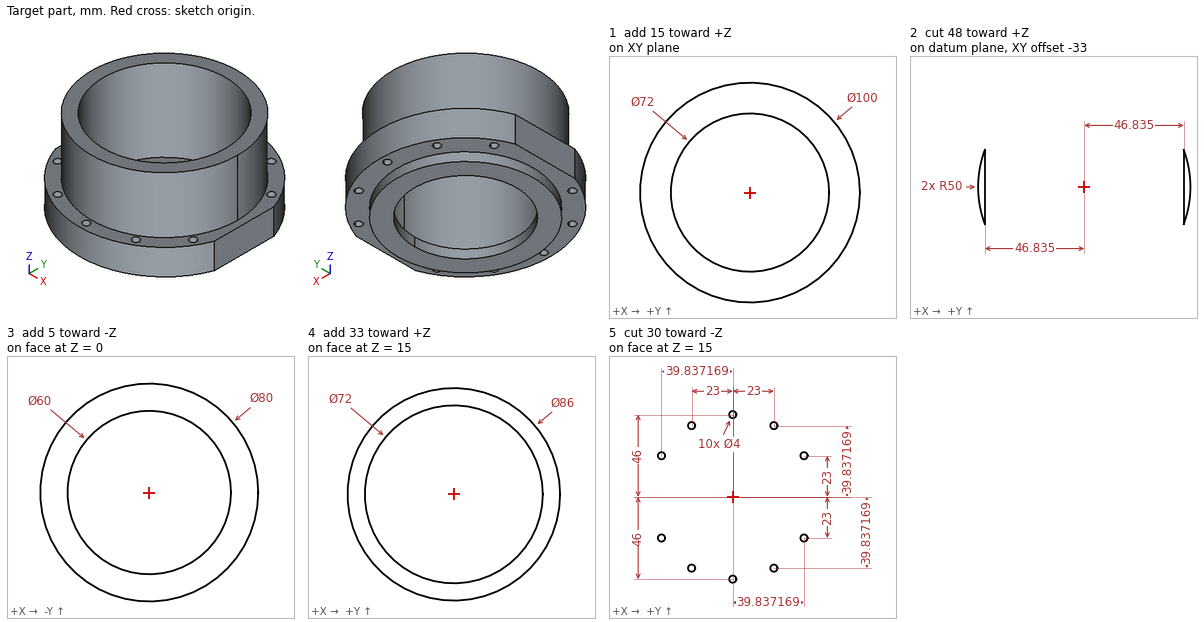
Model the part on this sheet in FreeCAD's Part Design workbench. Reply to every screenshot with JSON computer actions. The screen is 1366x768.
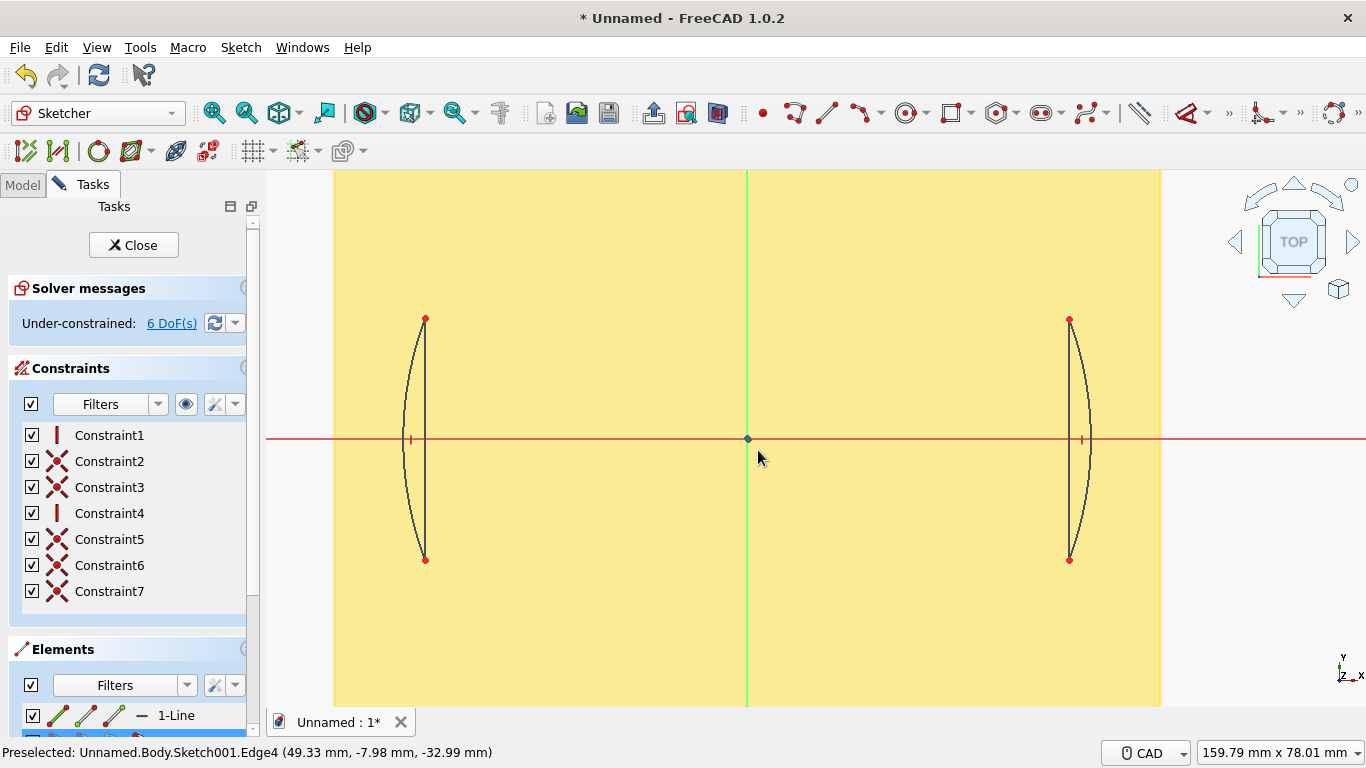
{"action": "key", "text": "c"}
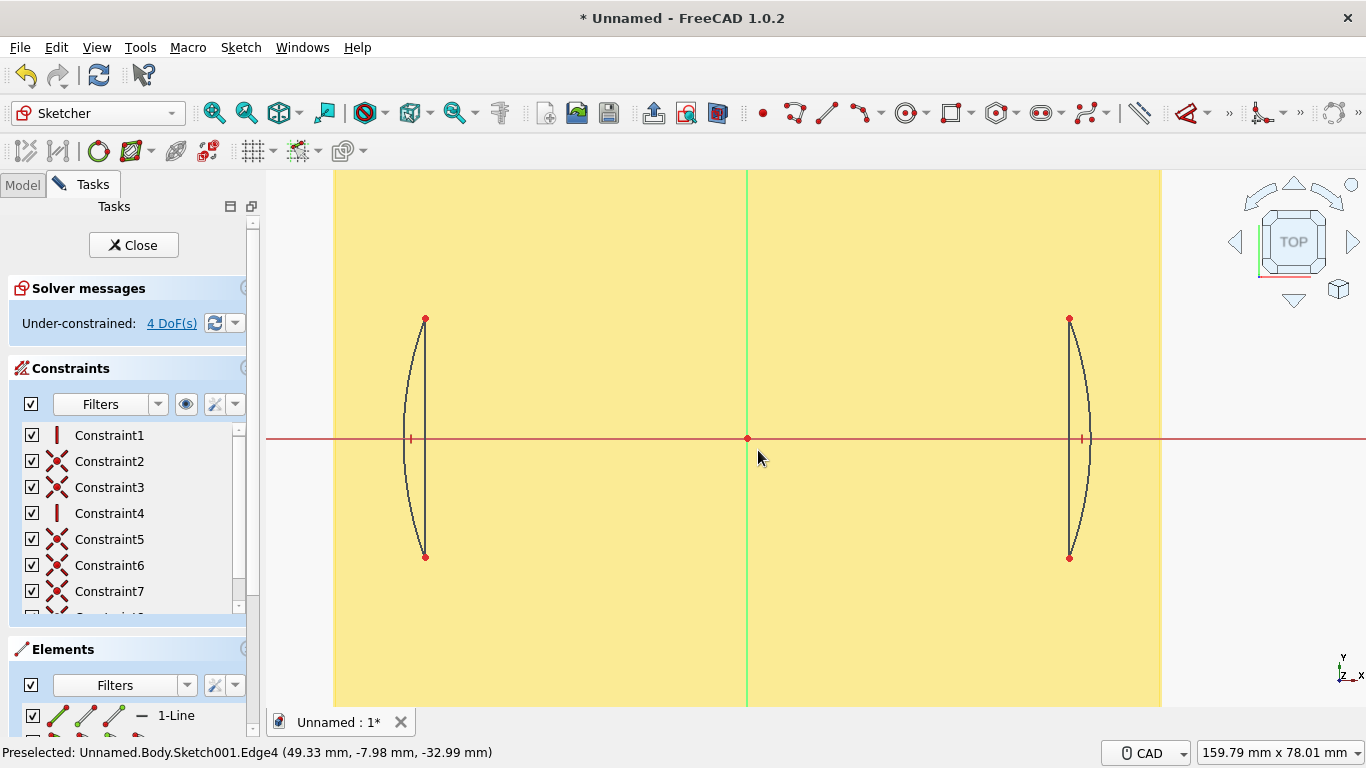
{"action": "left_click", "coordinate": [407, 390]}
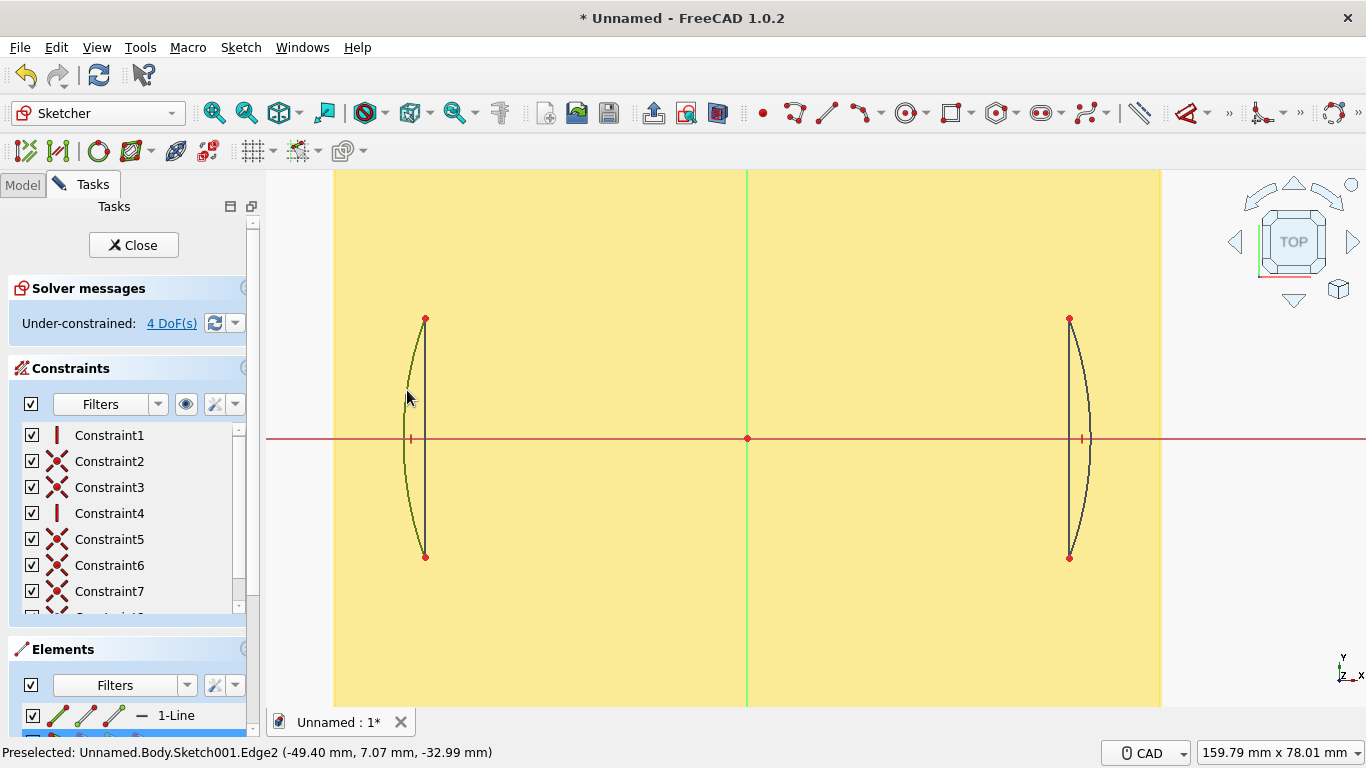
{"action": "left_click", "coordinate": [1087, 487]}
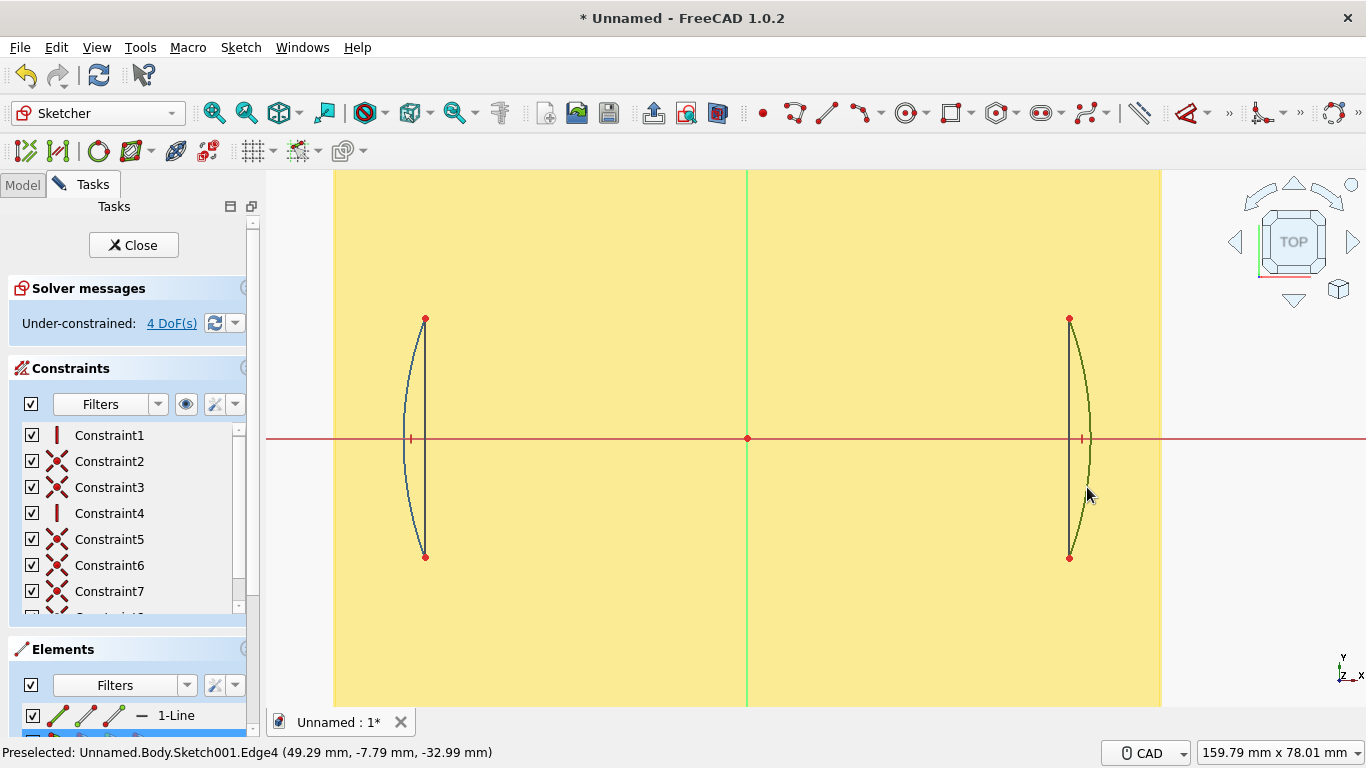
{"action": "key", "text": "e"}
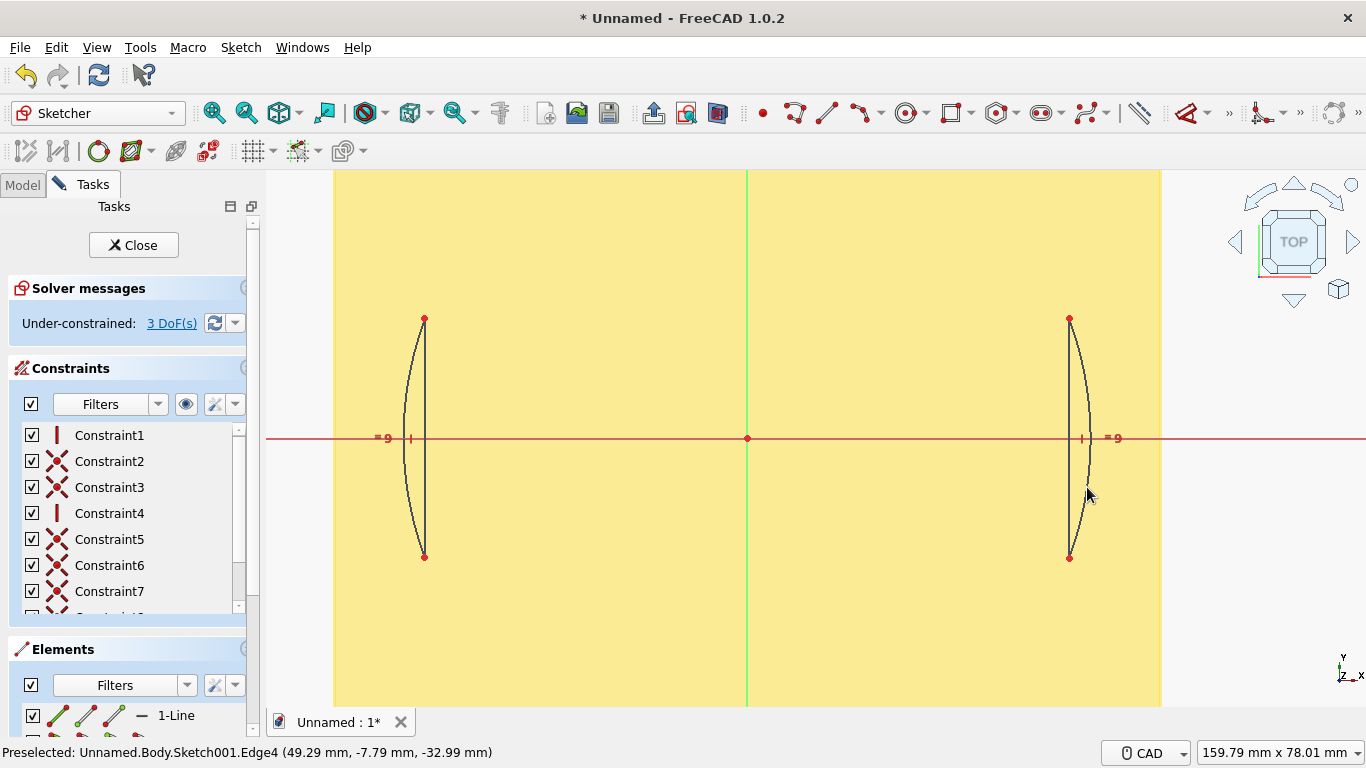
{"action": "left_click", "coordinate": [1186, 114]}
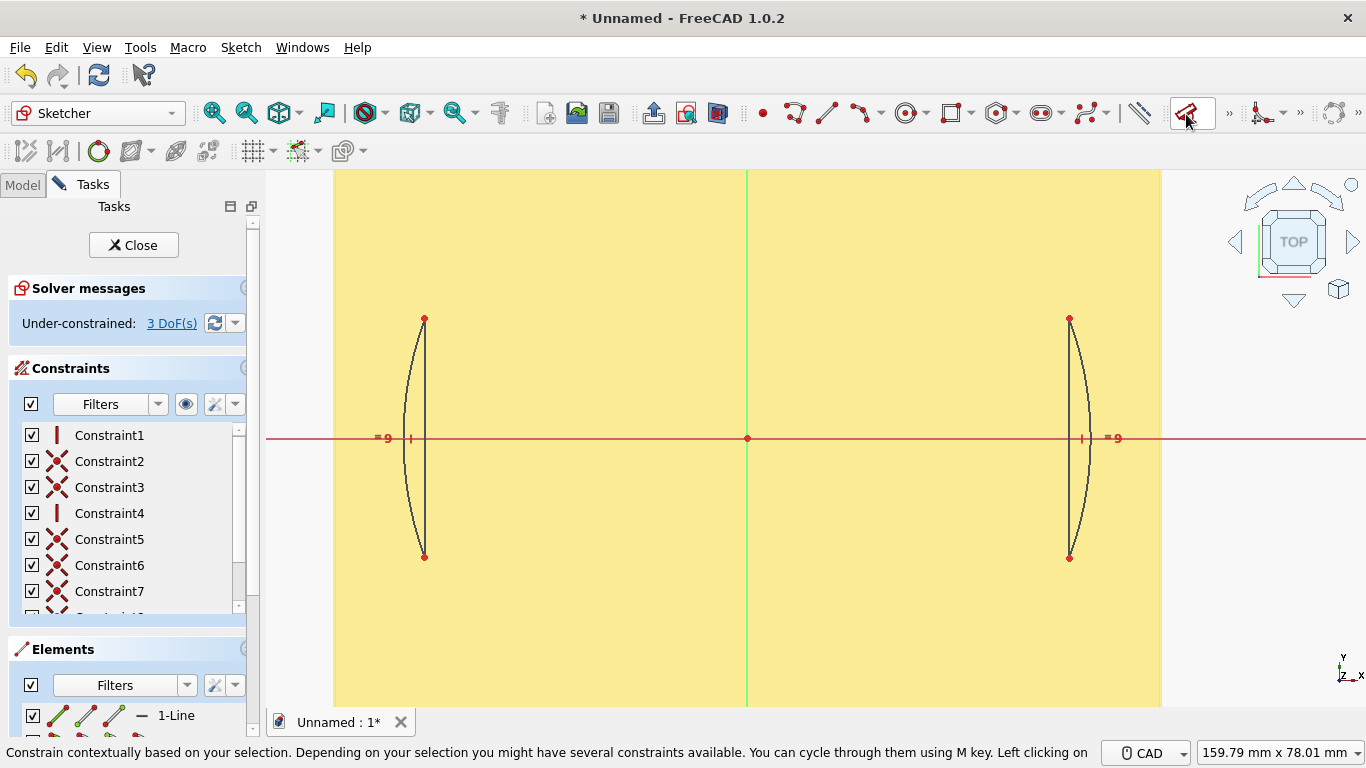
{"action": "left_click", "coordinate": [407, 390]}
{"action": "left_click", "coordinate": [375, 385]}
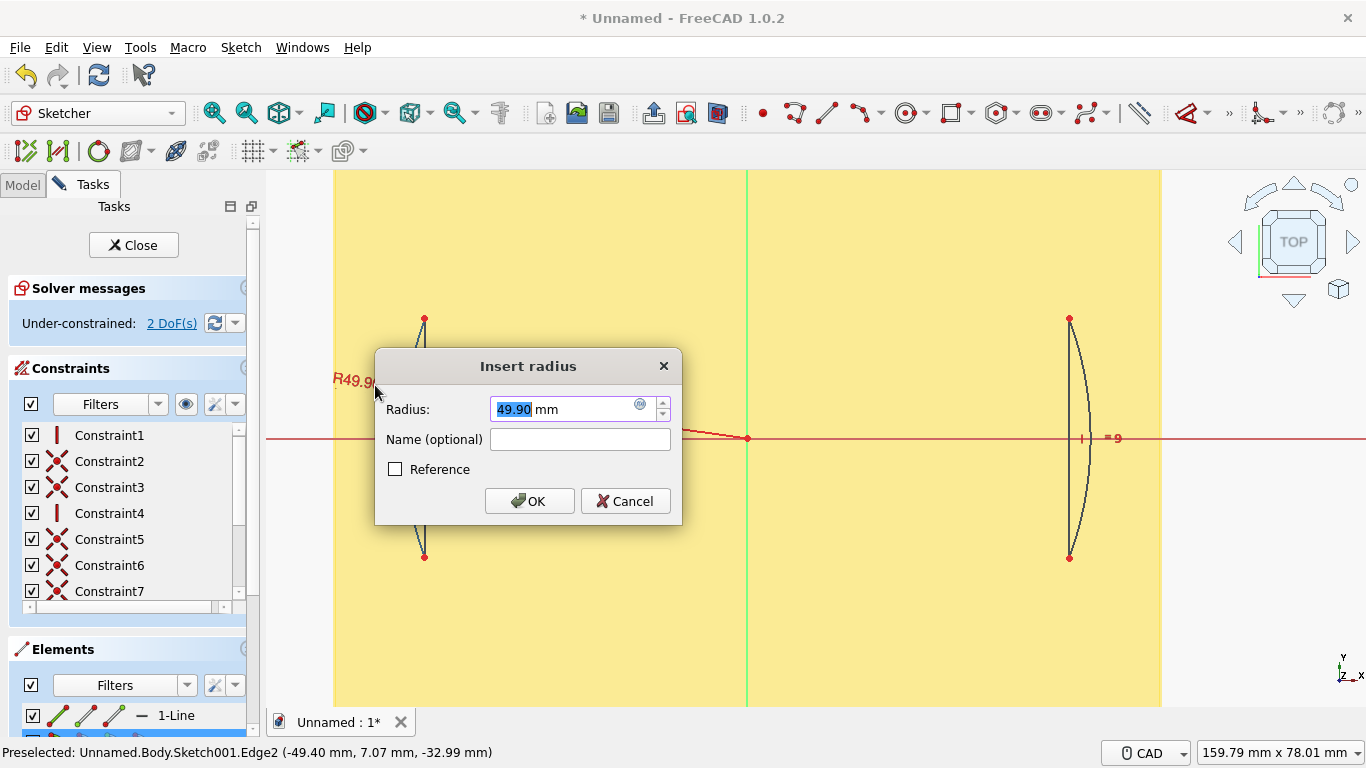
{"action": "type", "text": "50"}
{"action": "key", "text": "Return"}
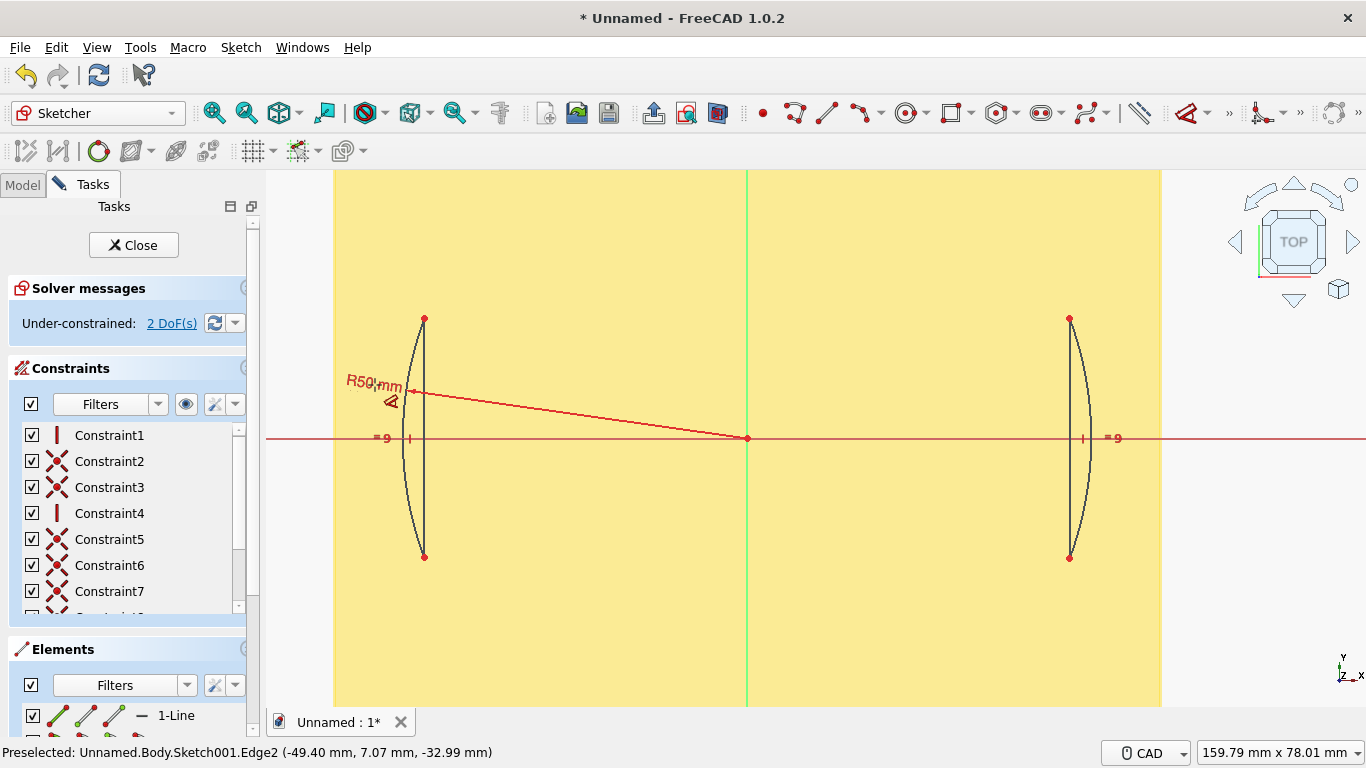
{"action": "left_click", "coordinate": [424, 558]}
{"action": "left_click", "coordinate": [586, 592]}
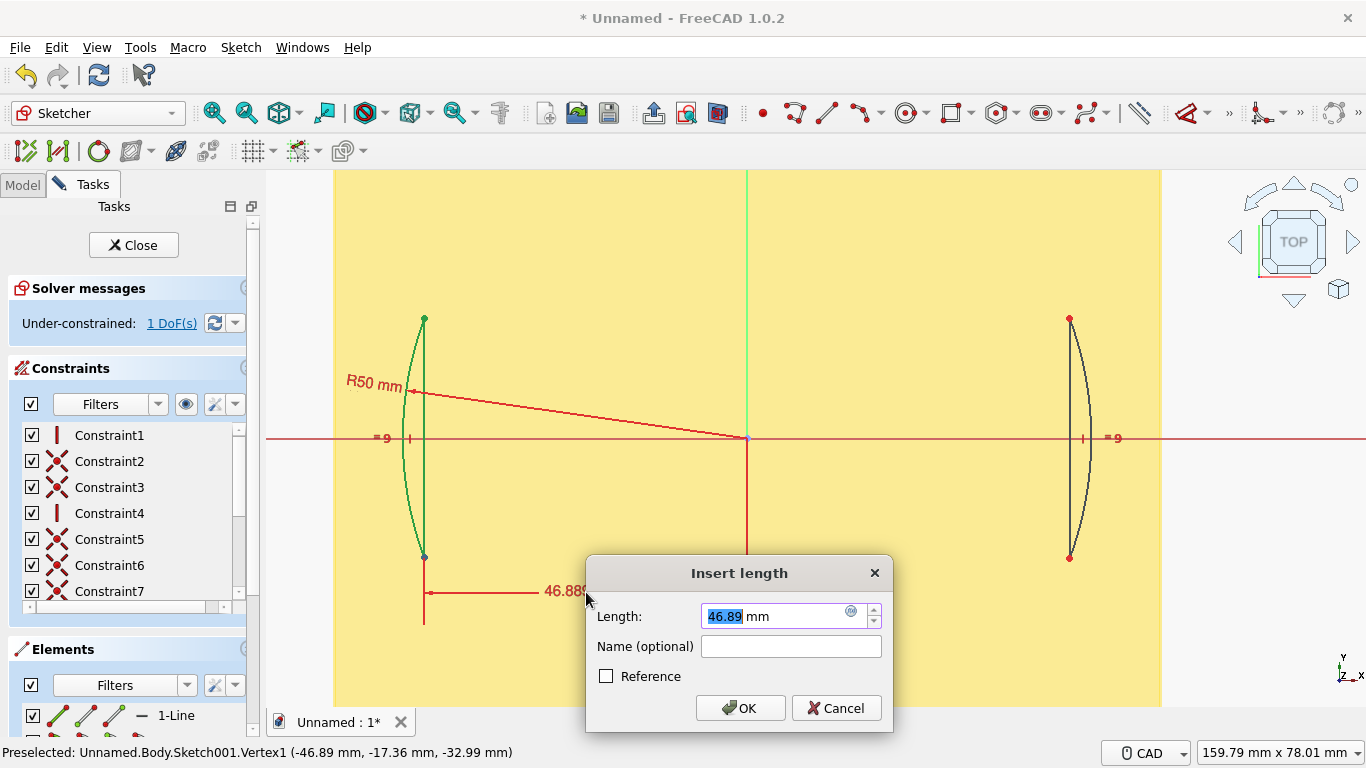
{"action": "type", "text": "46.835"}
{"action": "key", "text": "Return"}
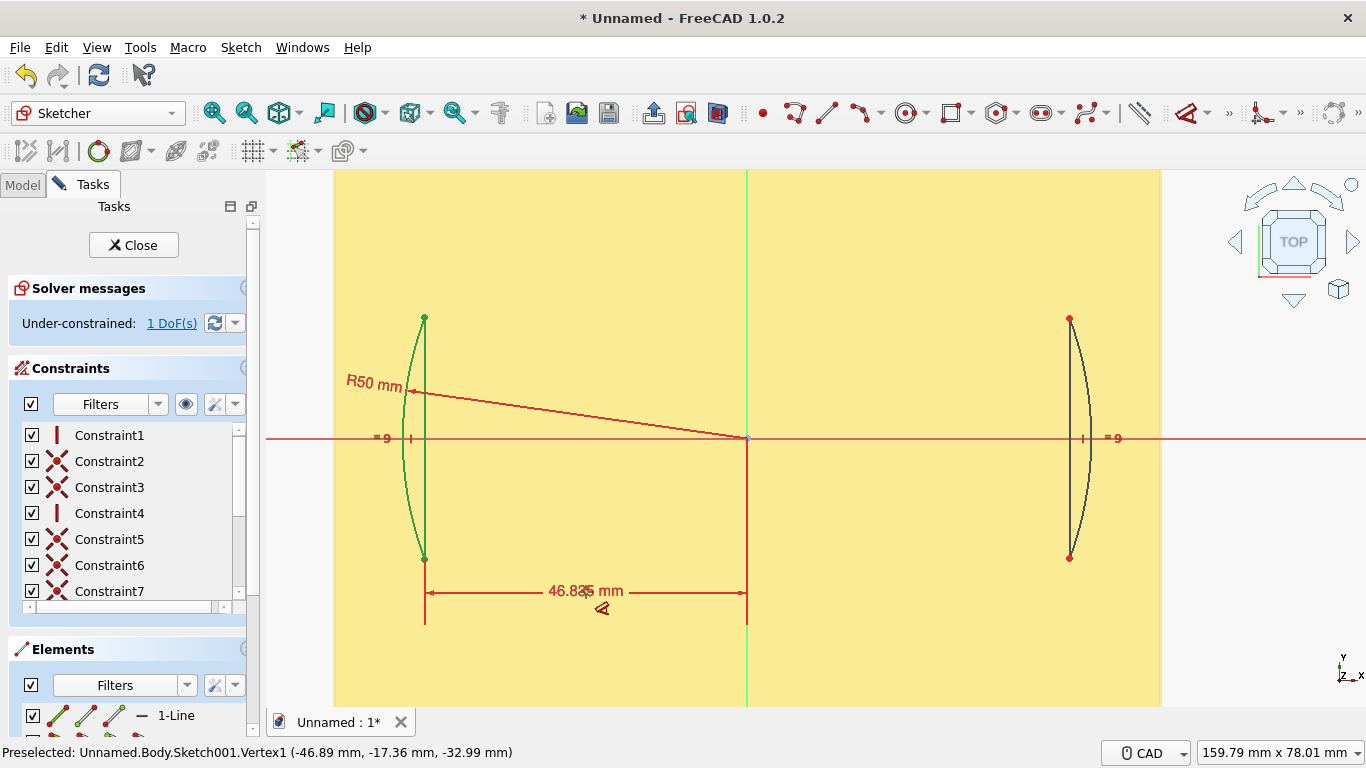
{"action": "left_click", "coordinate": [1070, 319]}
{"action": "left_click", "coordinate": [908, 285]}